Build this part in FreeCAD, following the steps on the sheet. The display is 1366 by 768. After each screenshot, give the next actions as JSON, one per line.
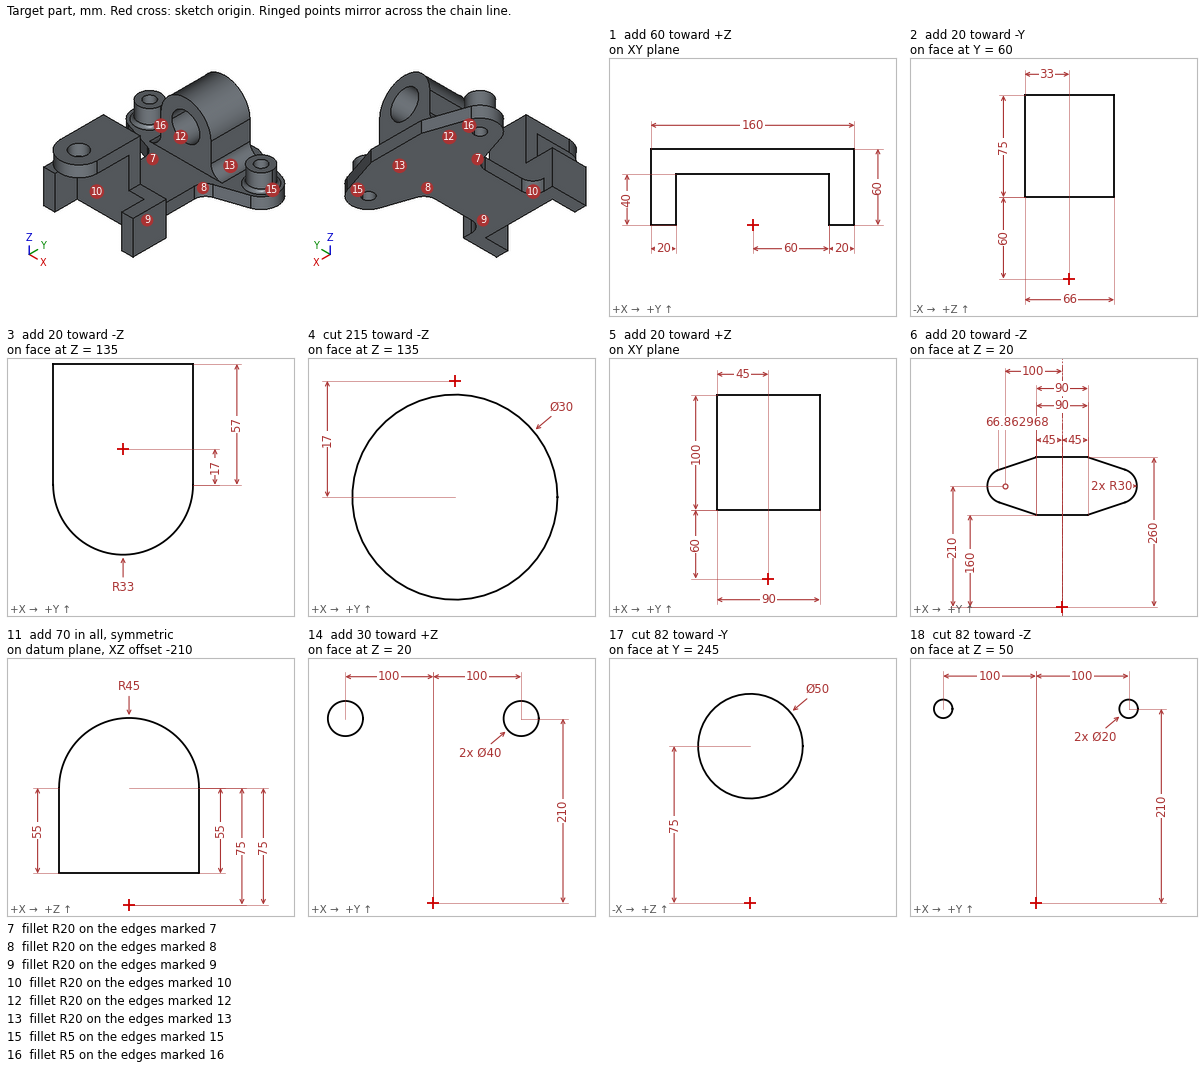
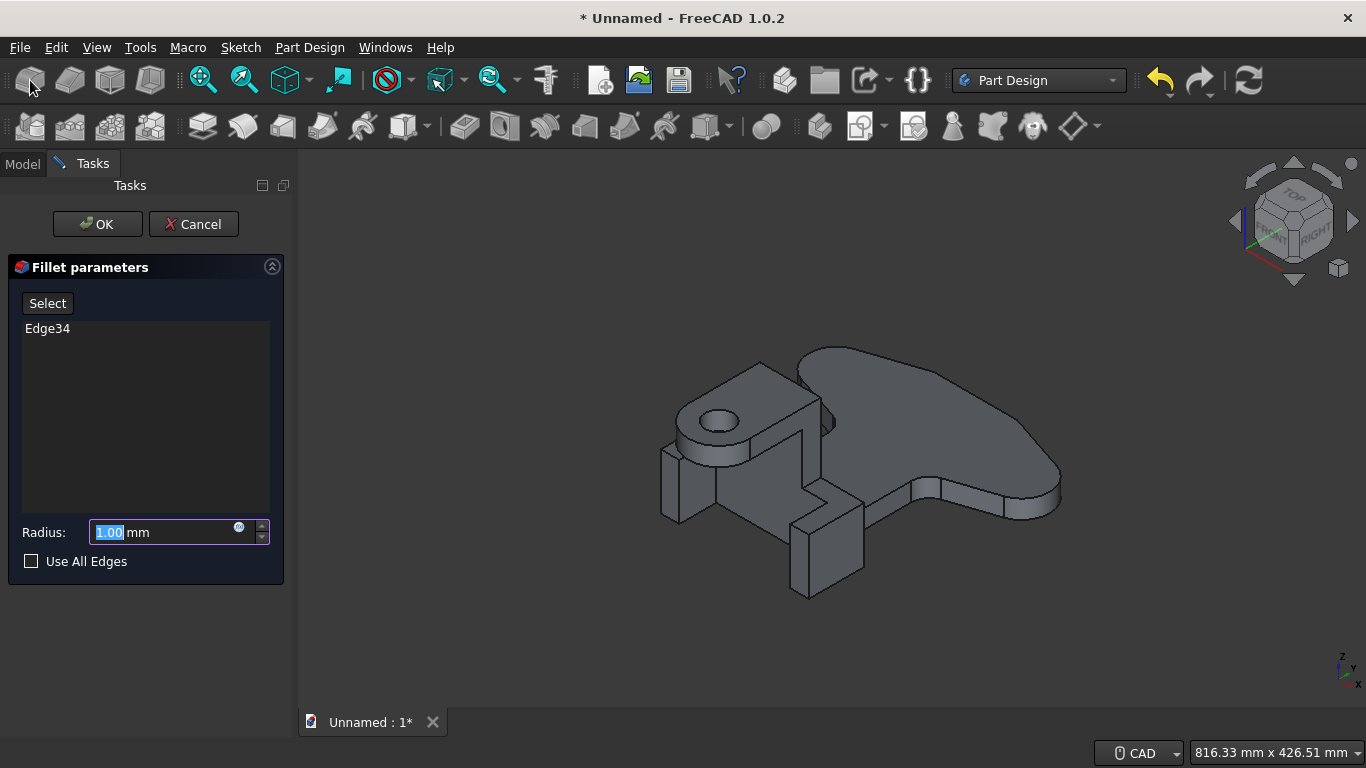
{"action": "type", "text": "20"}
{"action": "key", "text": "Tab"}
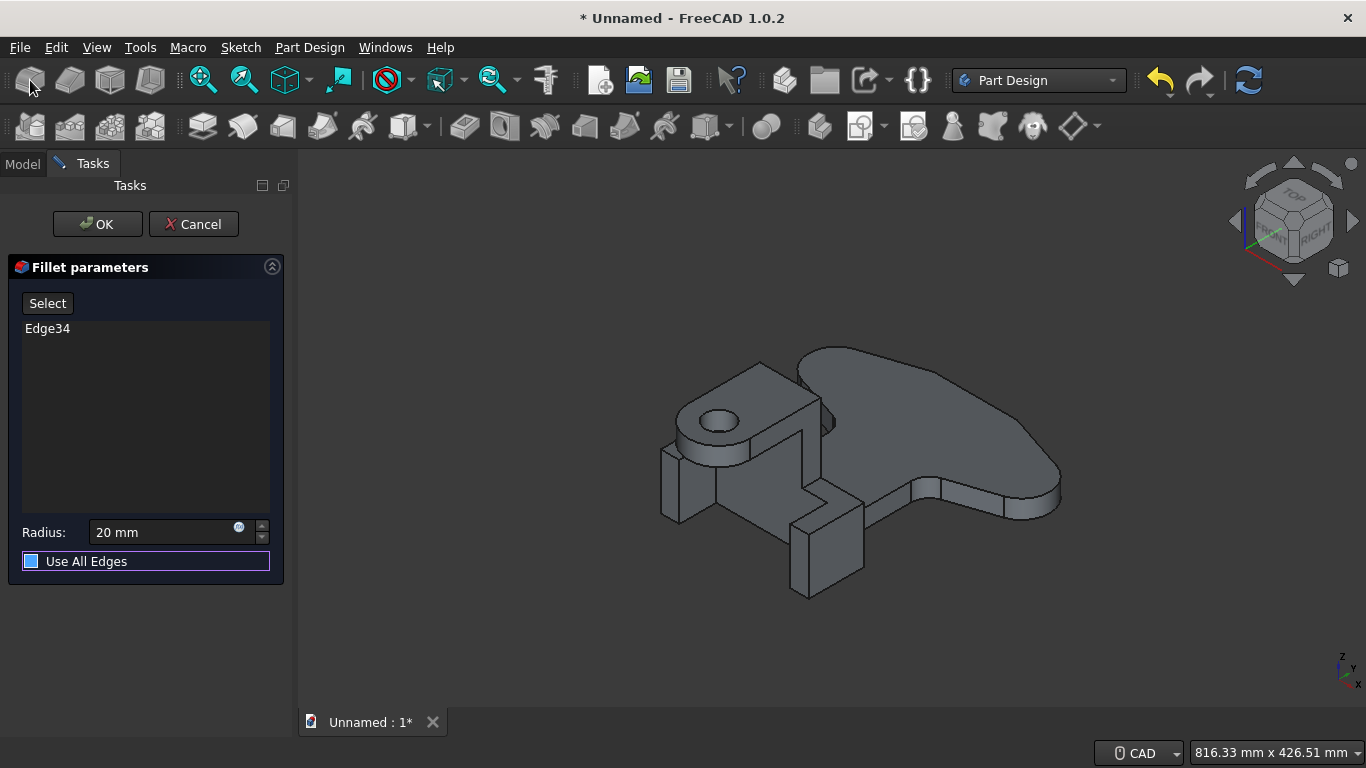
{"action": "left_click", "coordinate": [98, 224]}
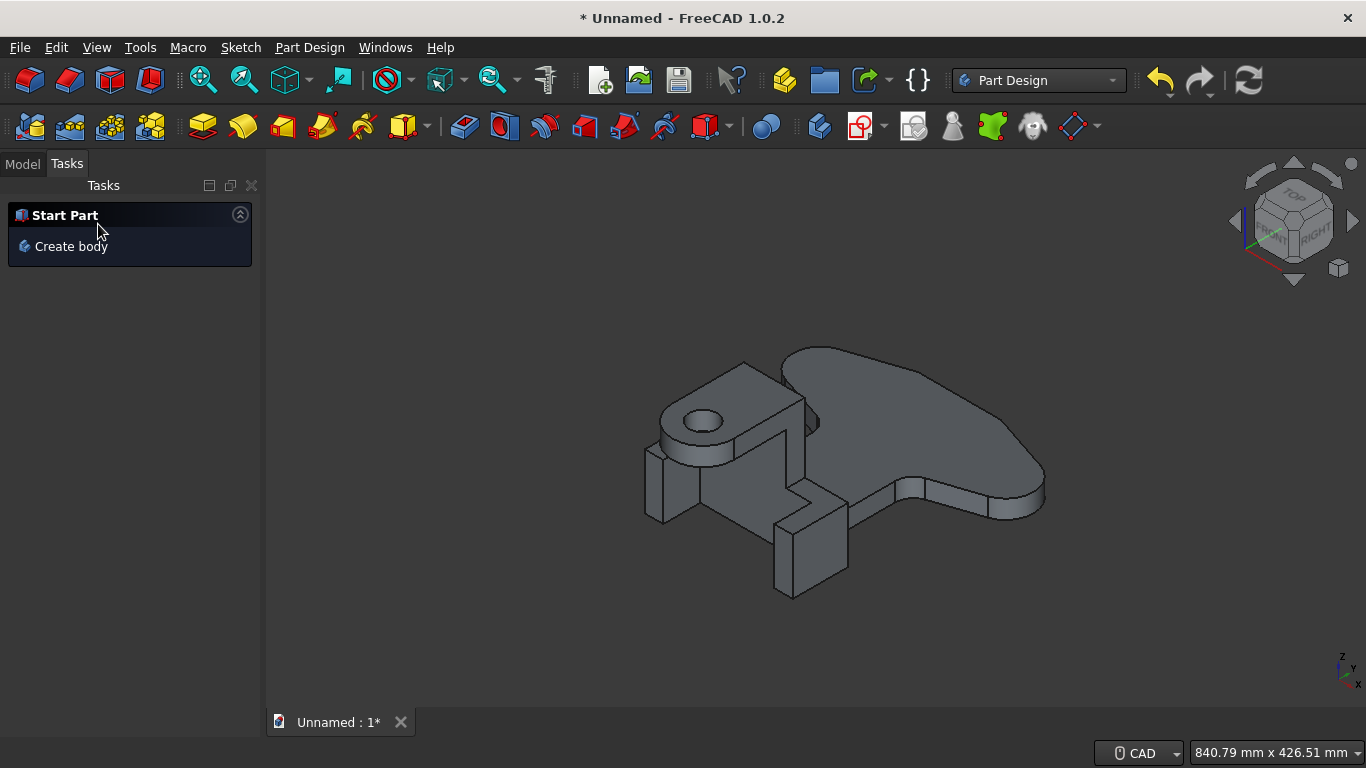
{"action": "left_click", "coordinate": [23, 163]}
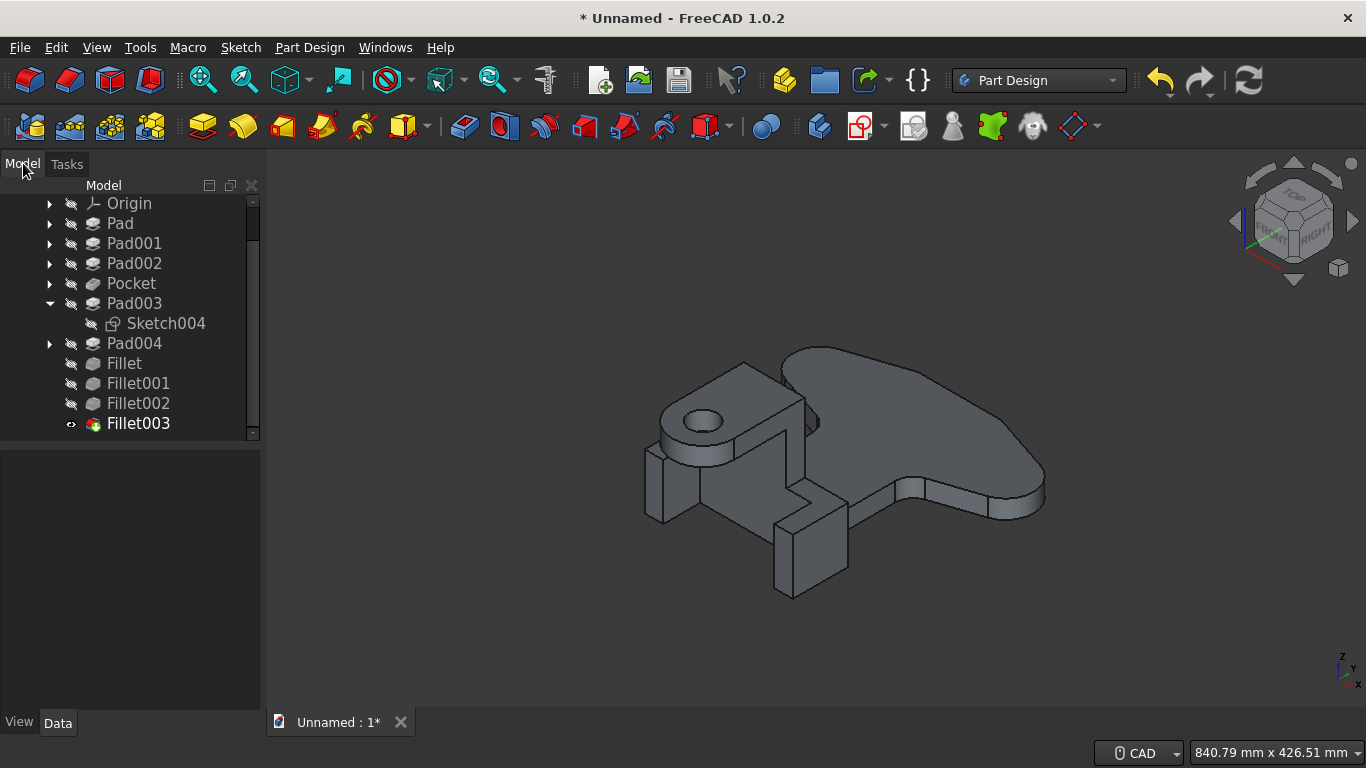
{"action": "left_click", "coordinate": [50, 204]}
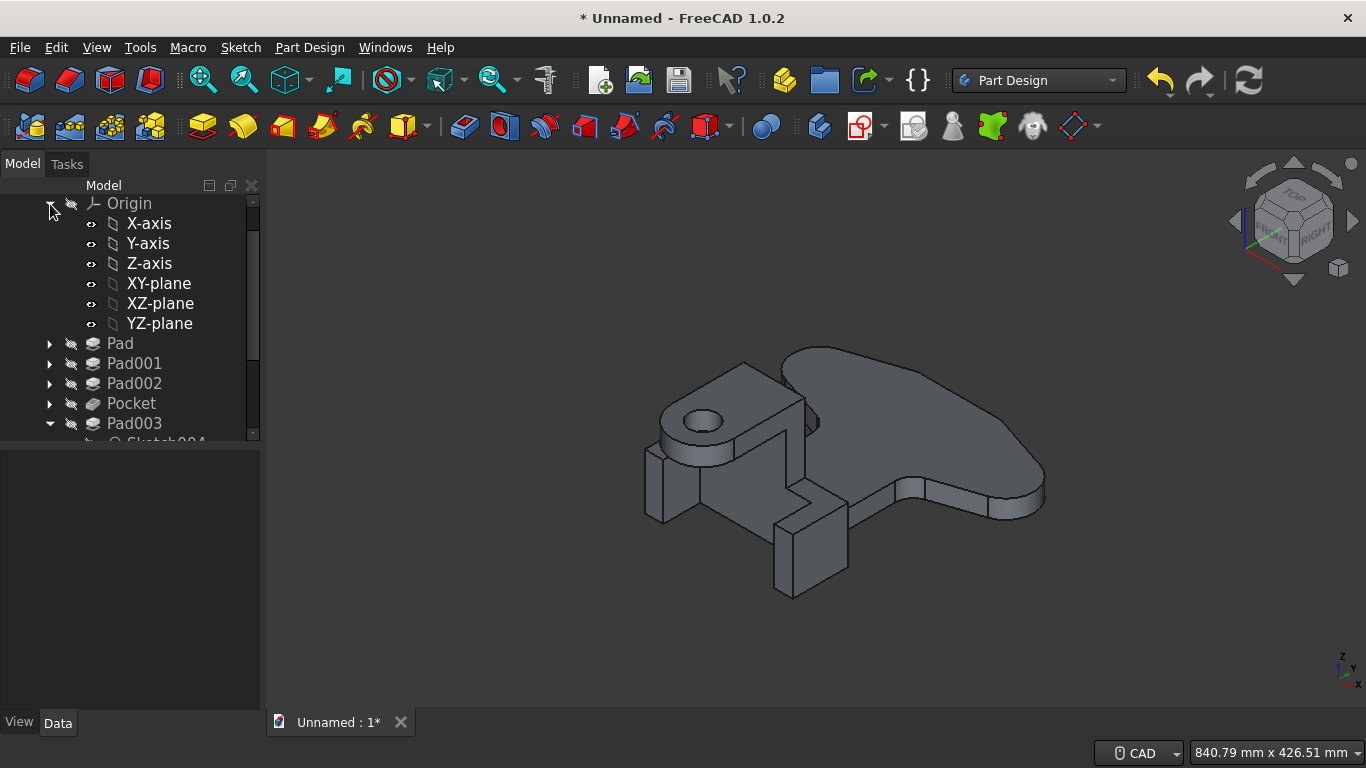
{"action": "left_click", "coordinate": [136, 304]}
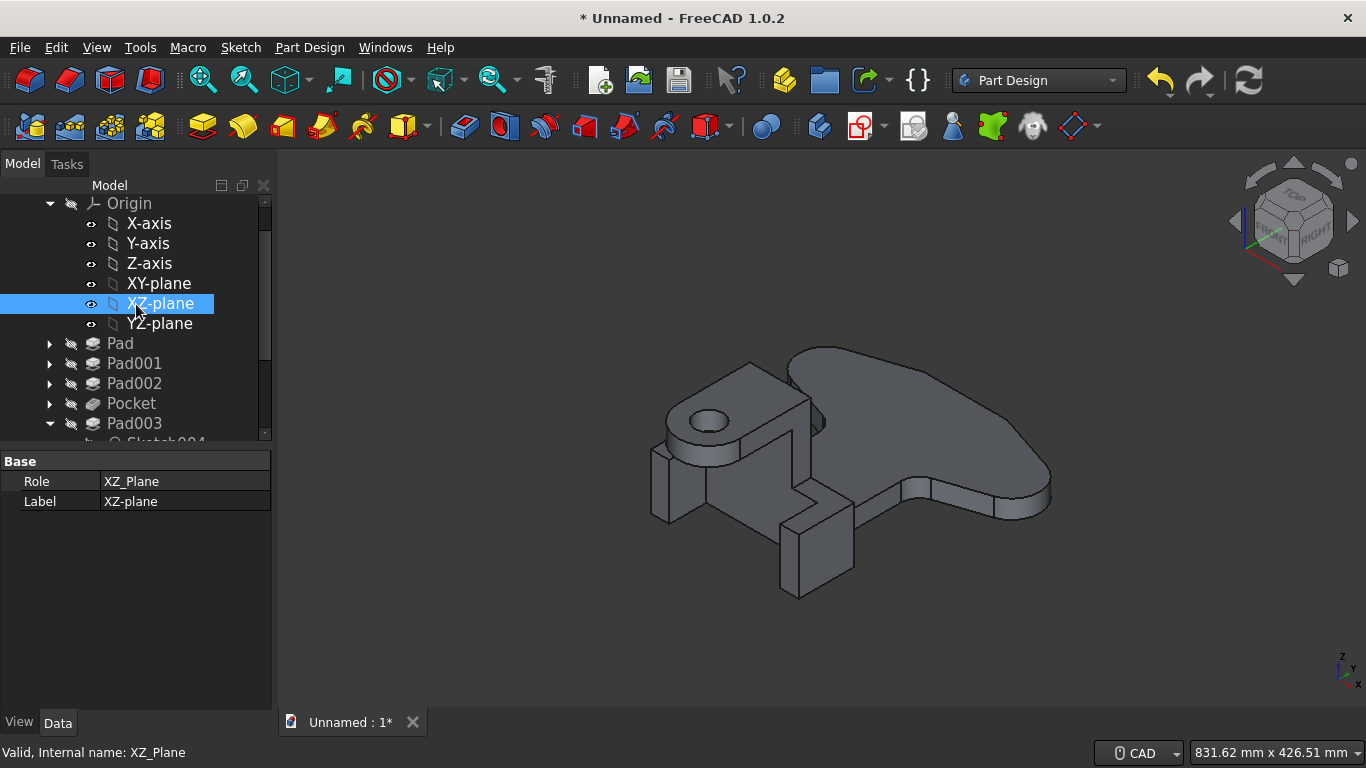
{"action": "left_click", "coordinate": [1074, 126]}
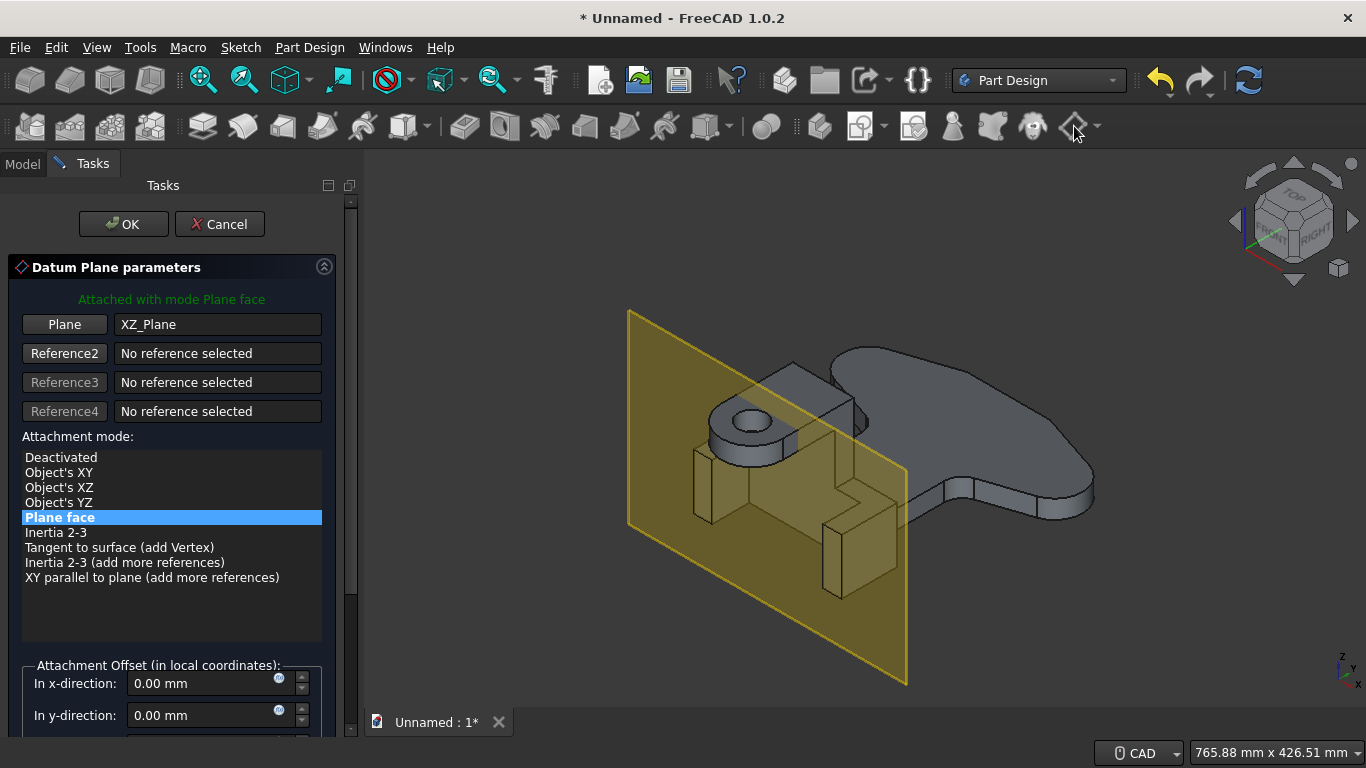
{"action": "scroll", "coordinate": [351, 466], "scroll_direction": "down", "scroll_amount": 2}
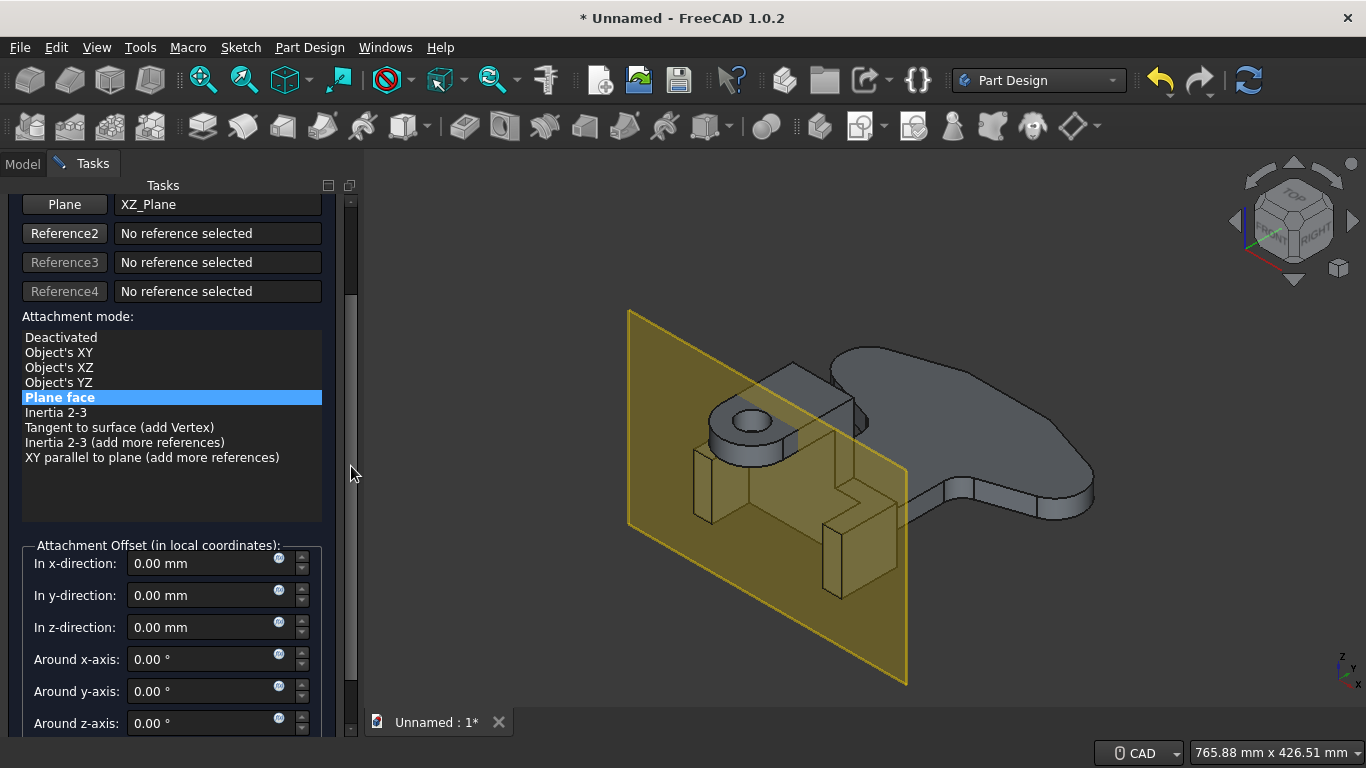
{"action": "triple_click", "coordinate": [210, 627]}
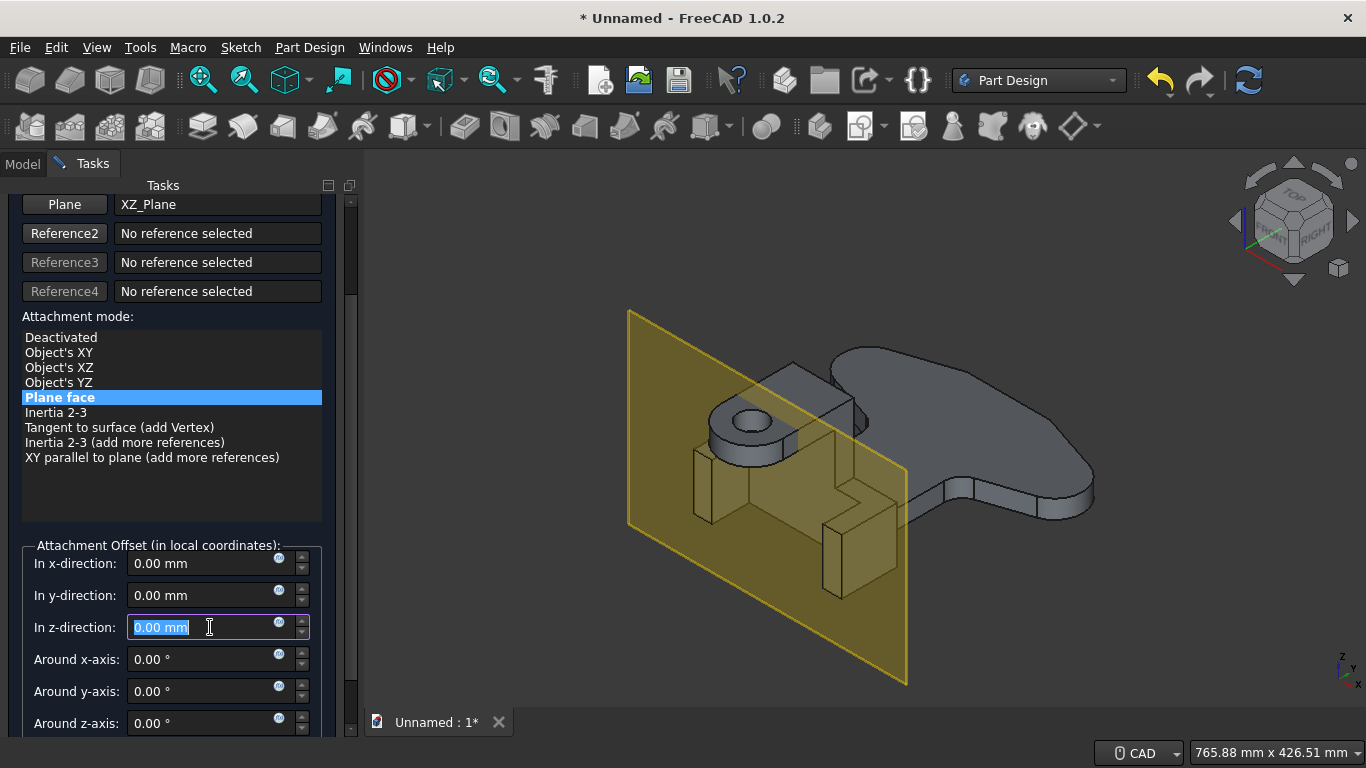
{"action": "type", "text": "-210"}
{"action": "key", "text": "Tab"}